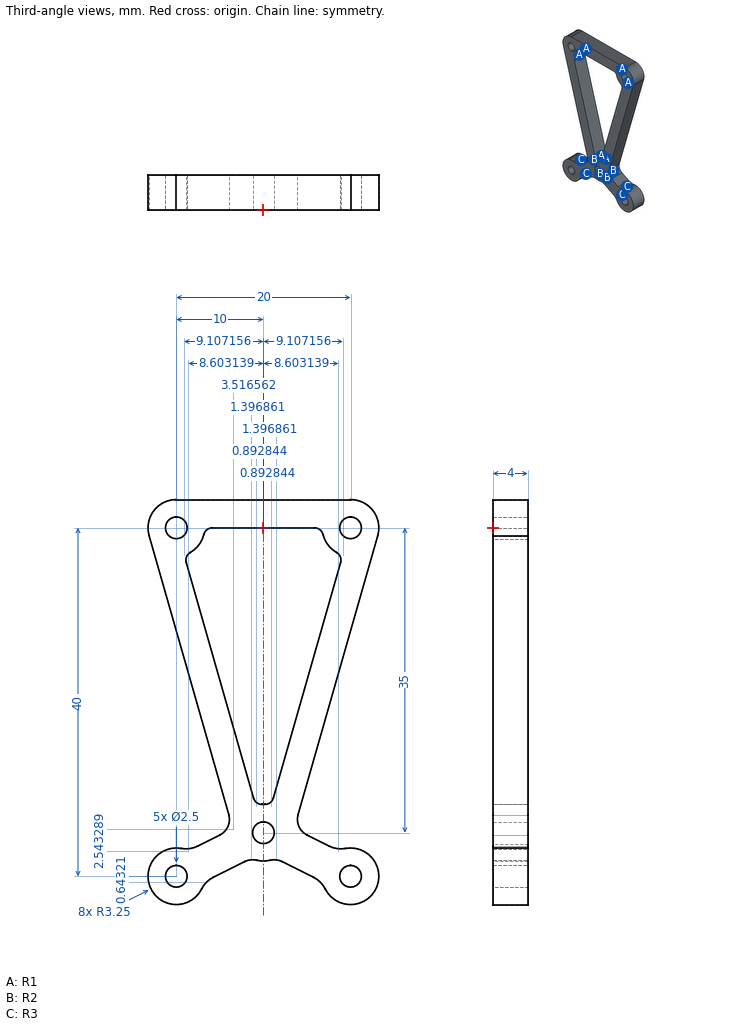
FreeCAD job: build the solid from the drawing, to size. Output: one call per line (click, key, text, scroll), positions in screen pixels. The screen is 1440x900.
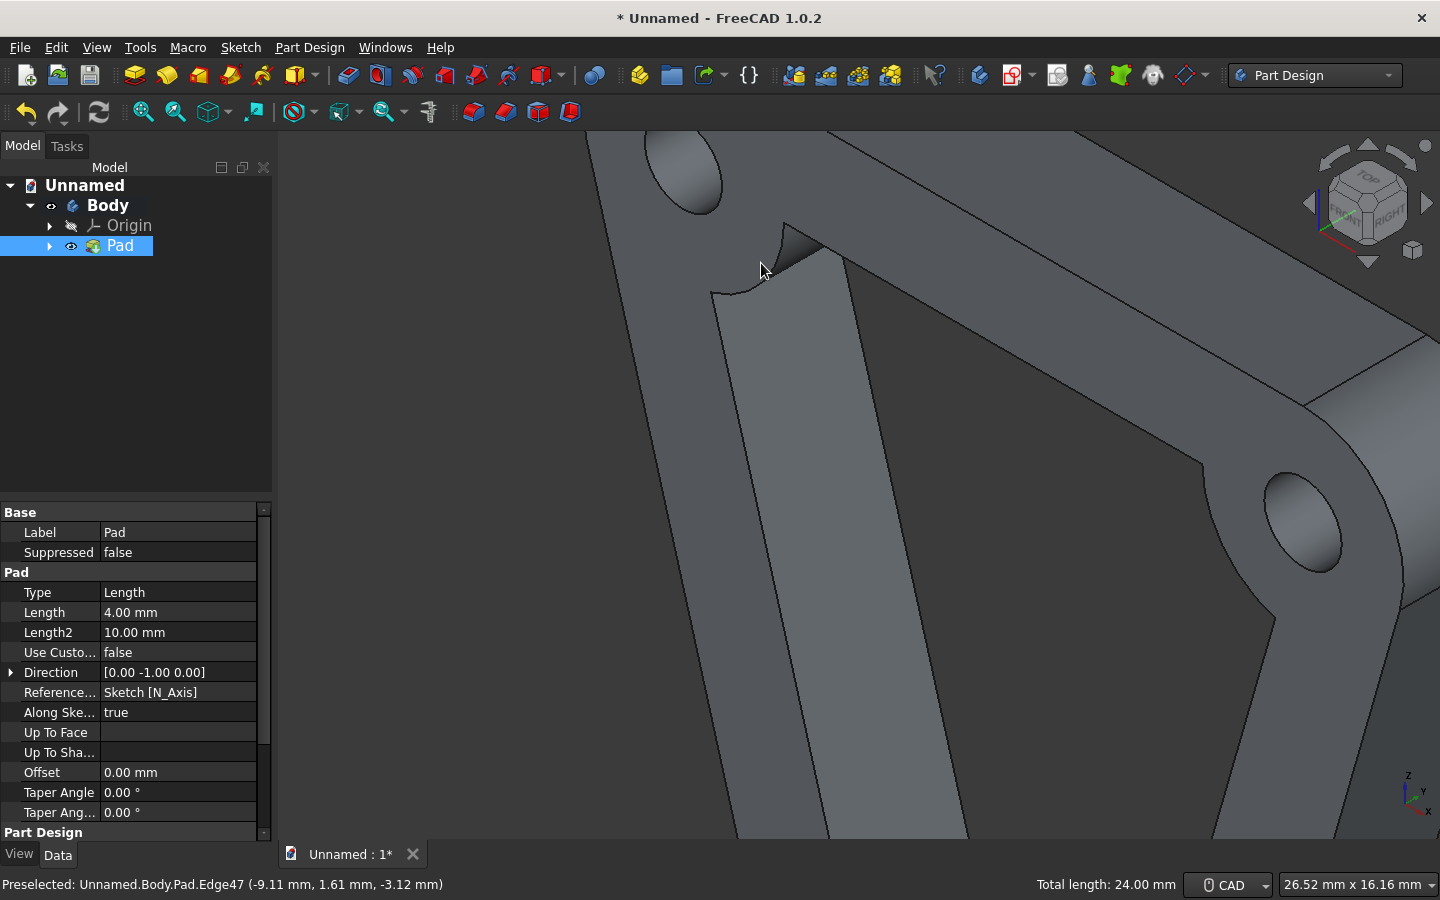
click(474, 112)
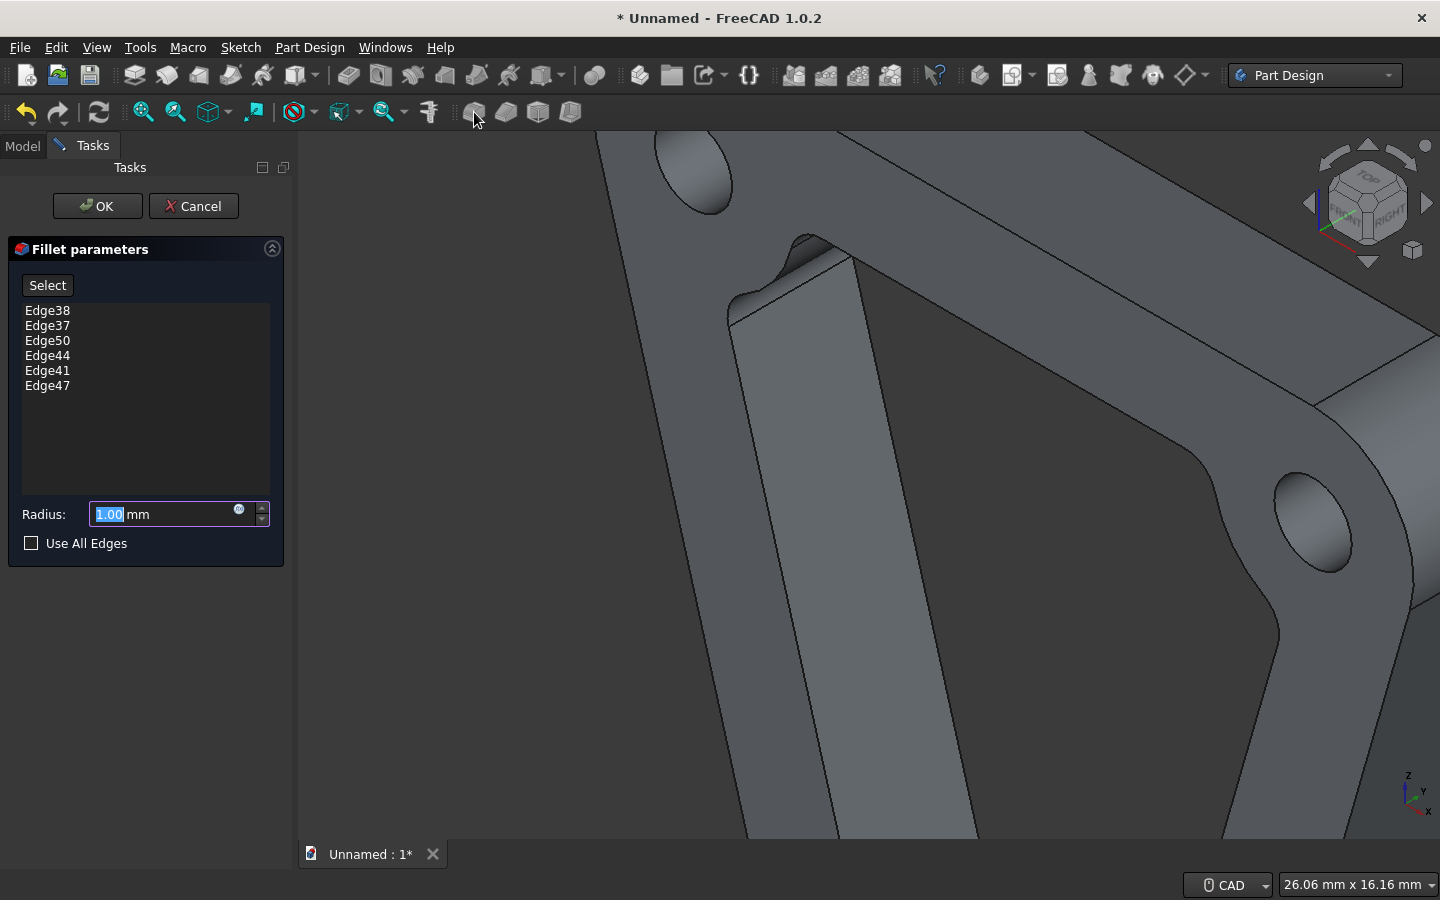
text(1)
key(Tab)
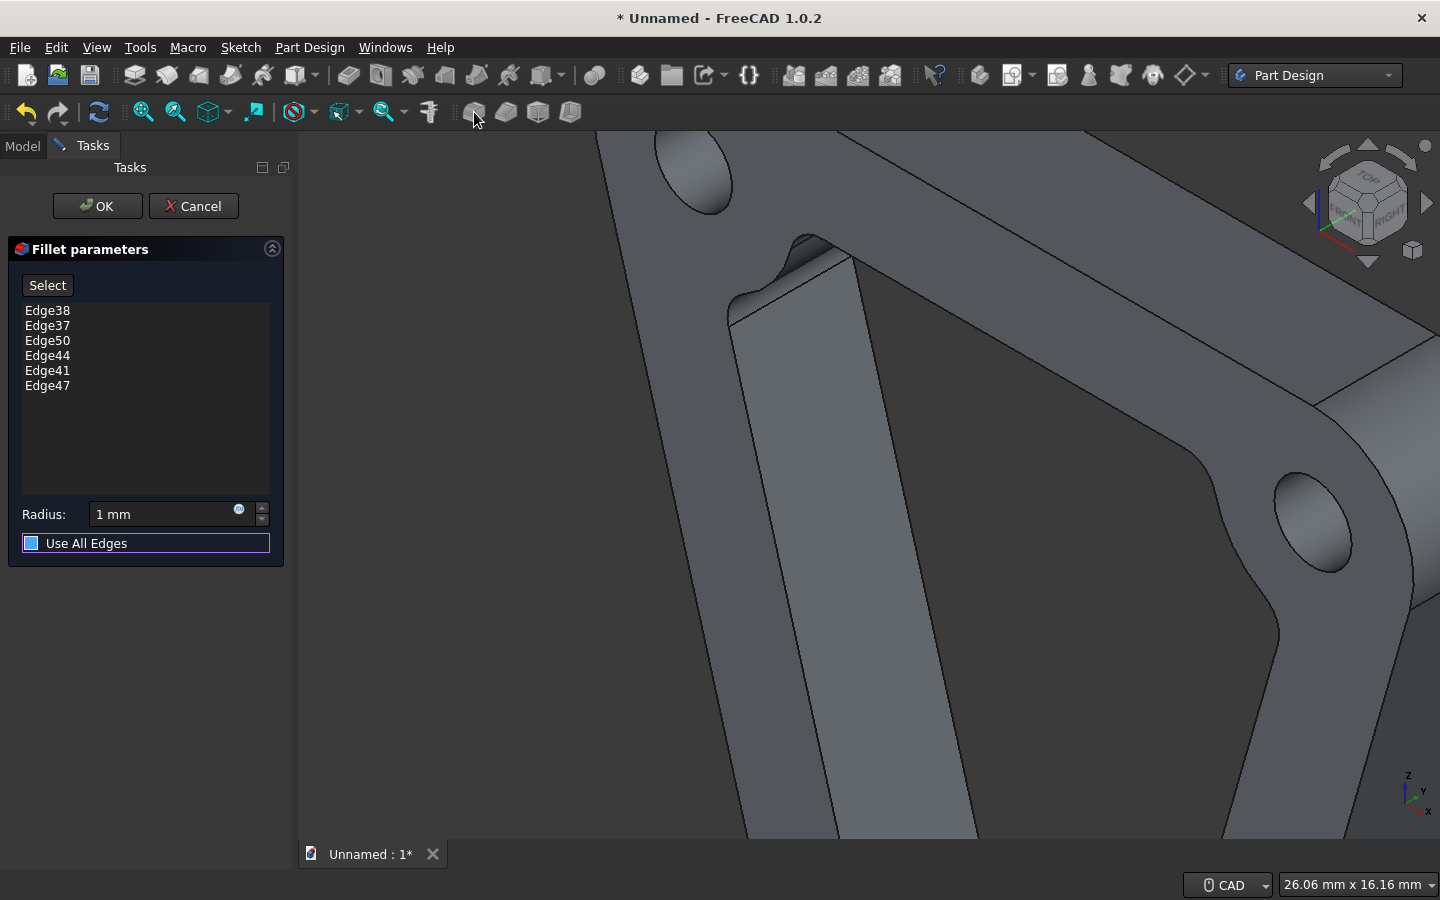
click(98, 206)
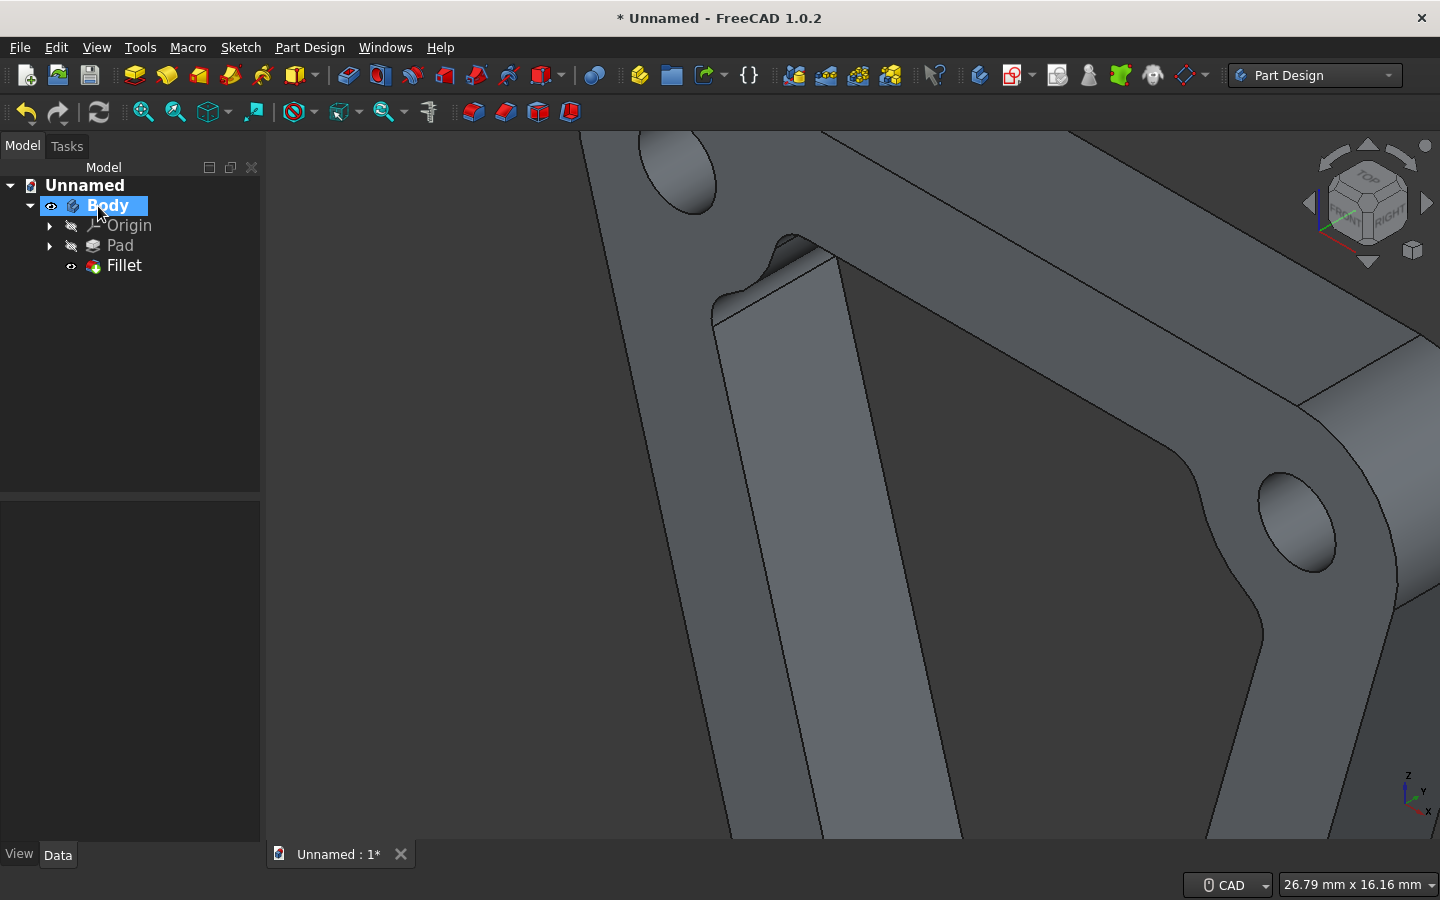
click(144, 112)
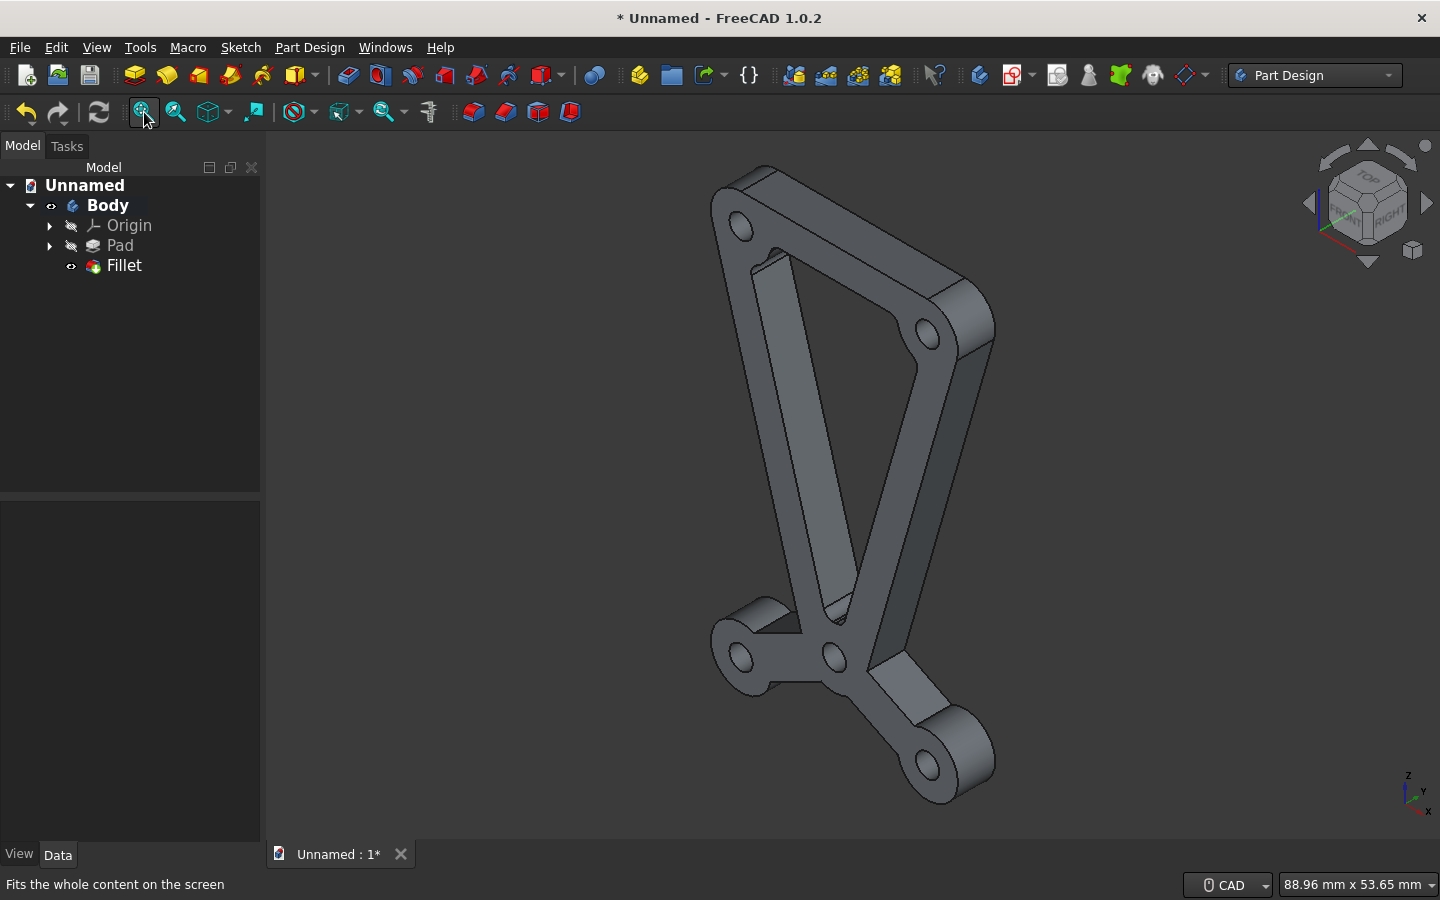
key(2)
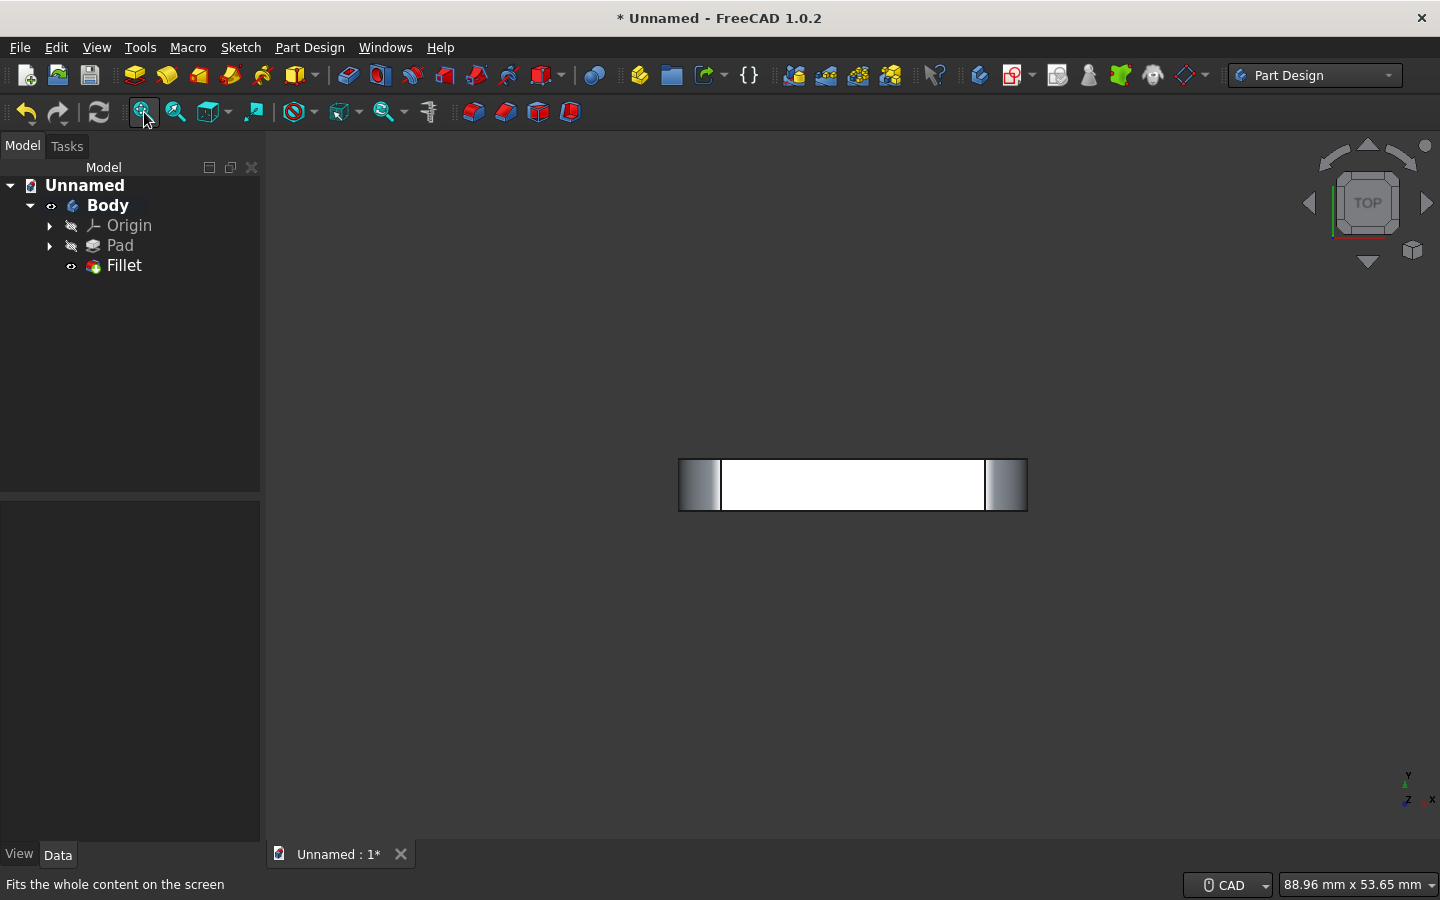
click(144, 112)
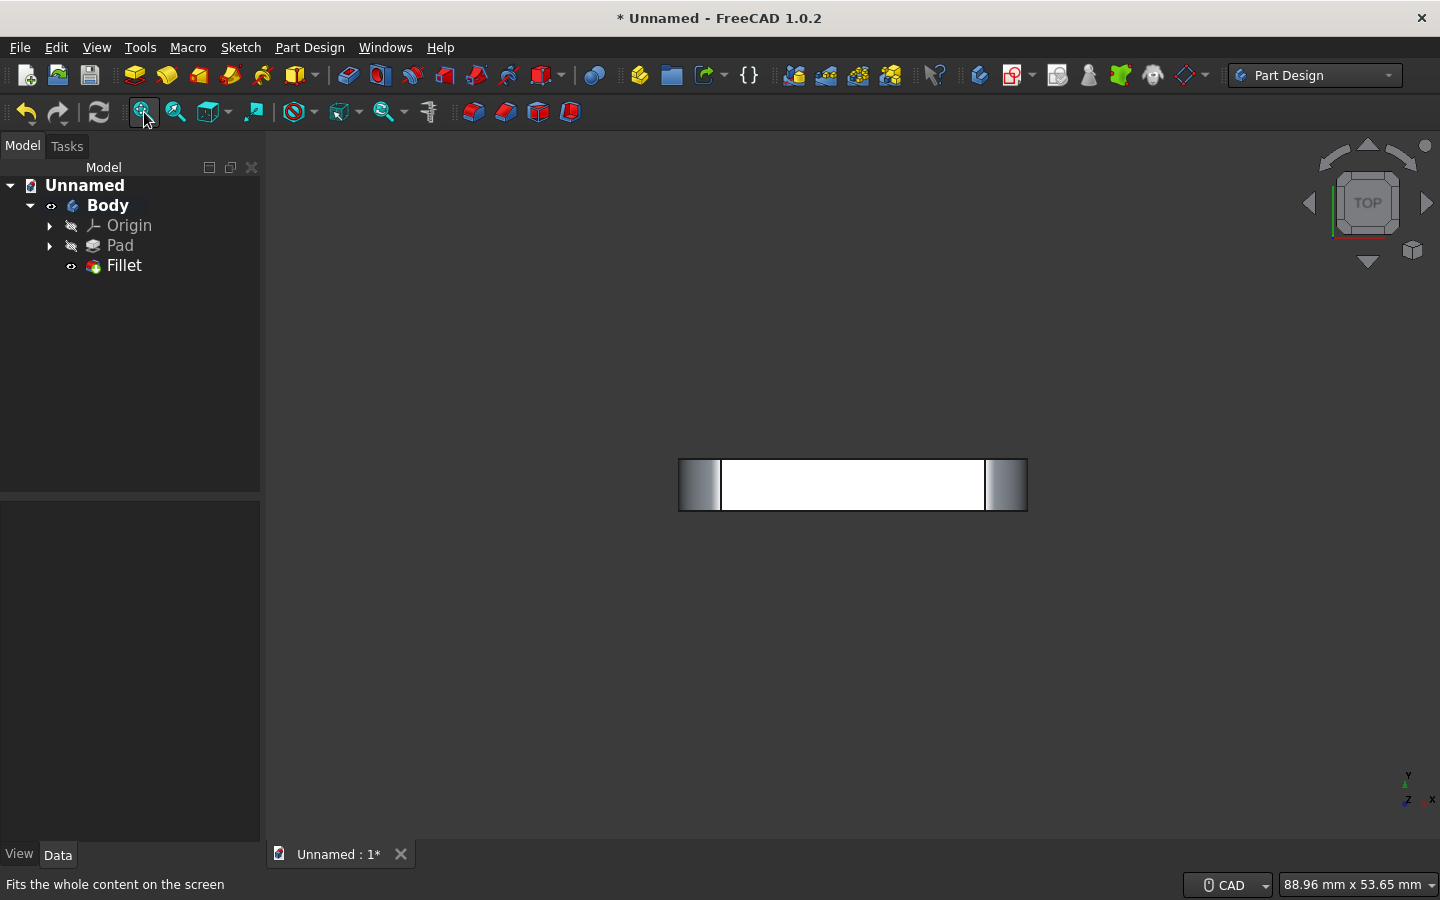
key(0)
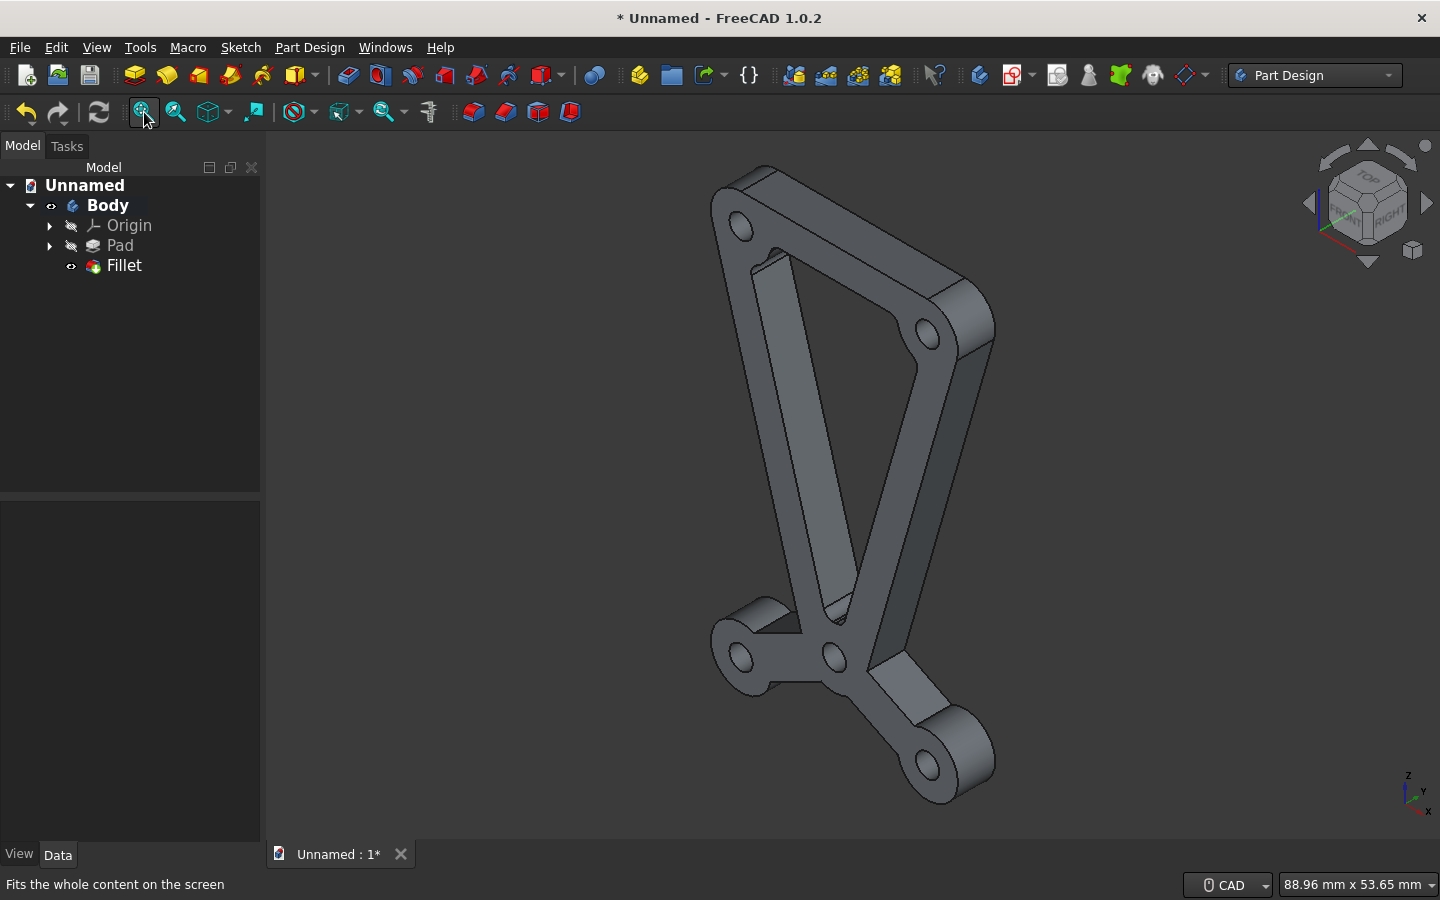
key(1)